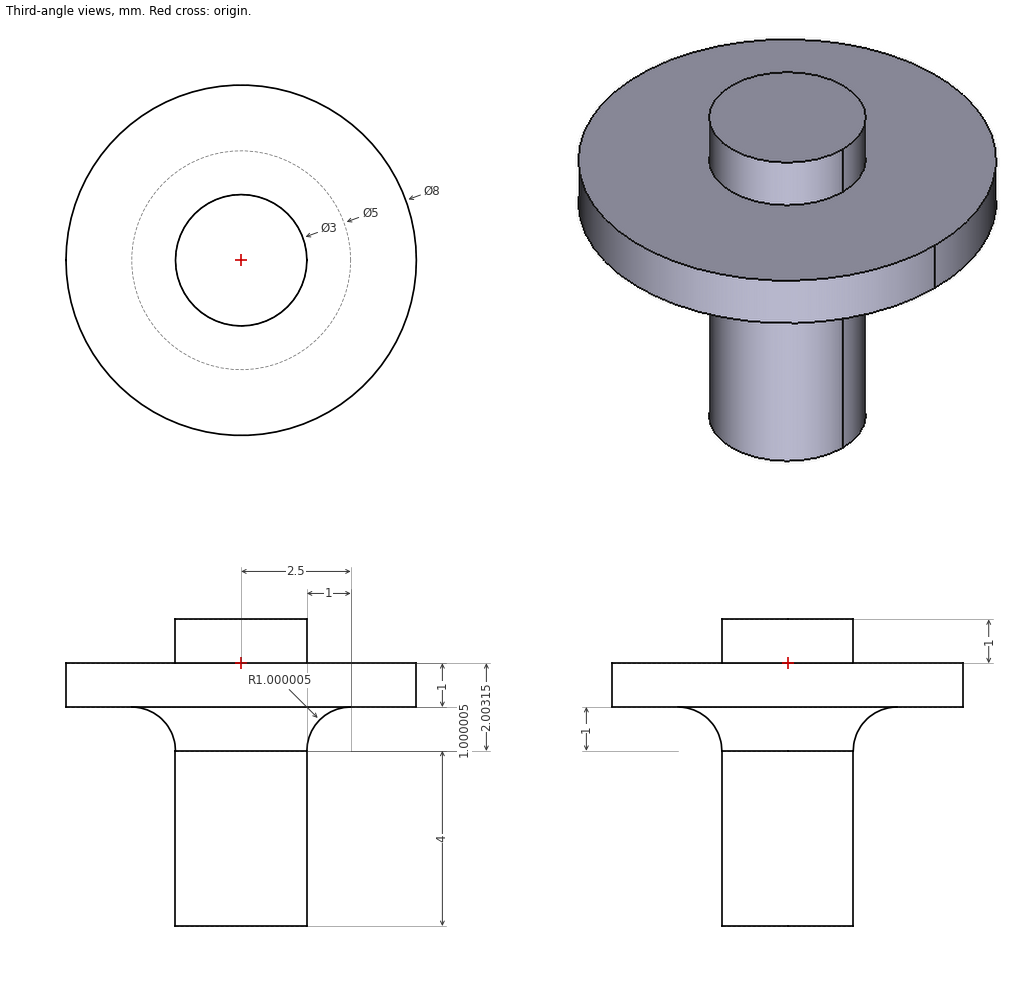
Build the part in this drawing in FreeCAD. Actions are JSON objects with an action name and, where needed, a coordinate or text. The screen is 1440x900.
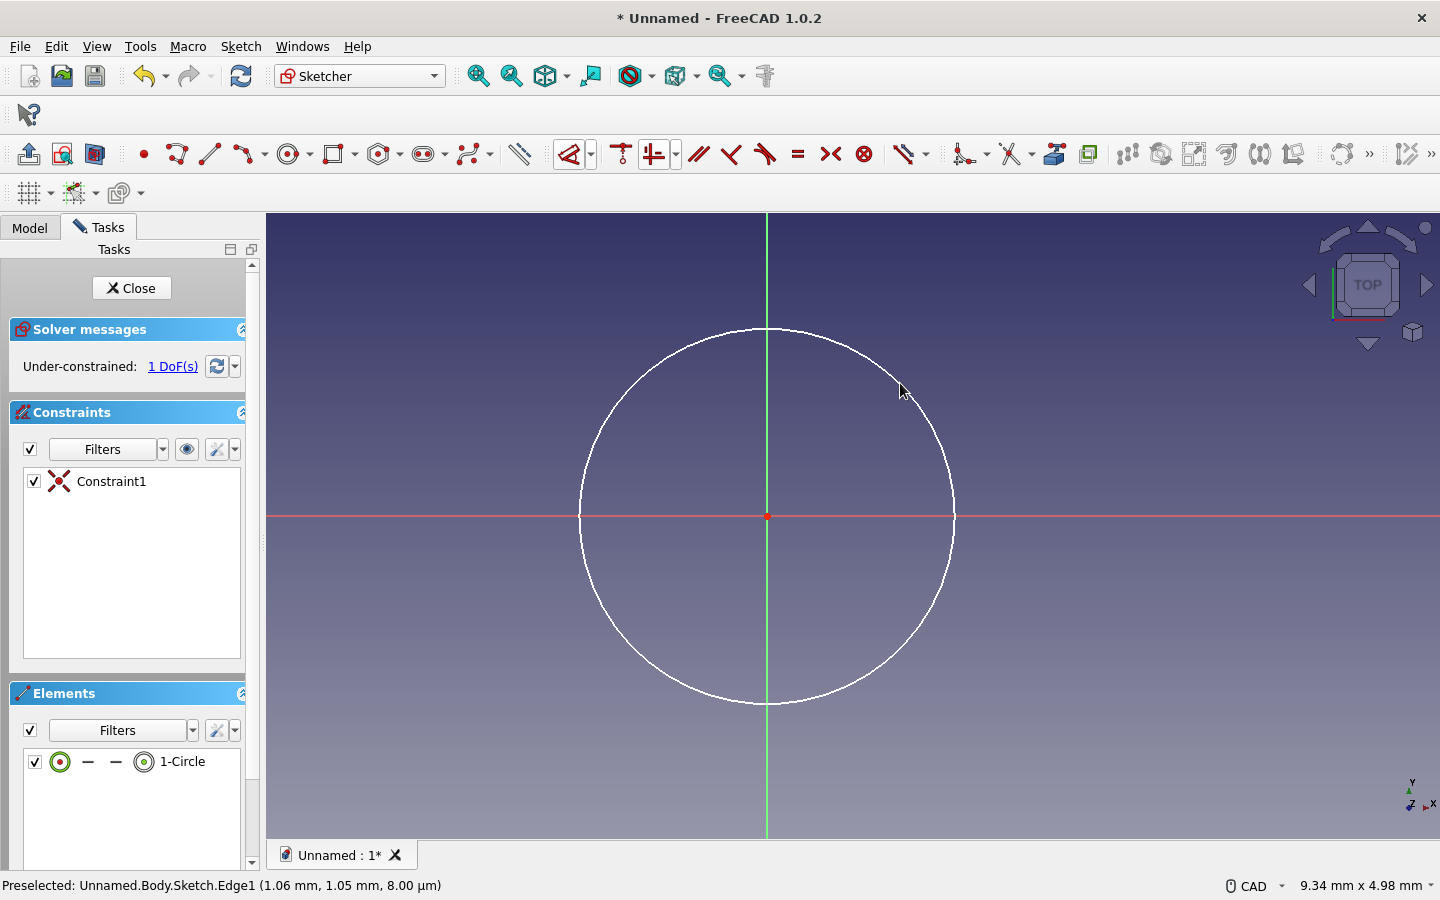
{"action": "left_click", "coordinate": [899, 383]}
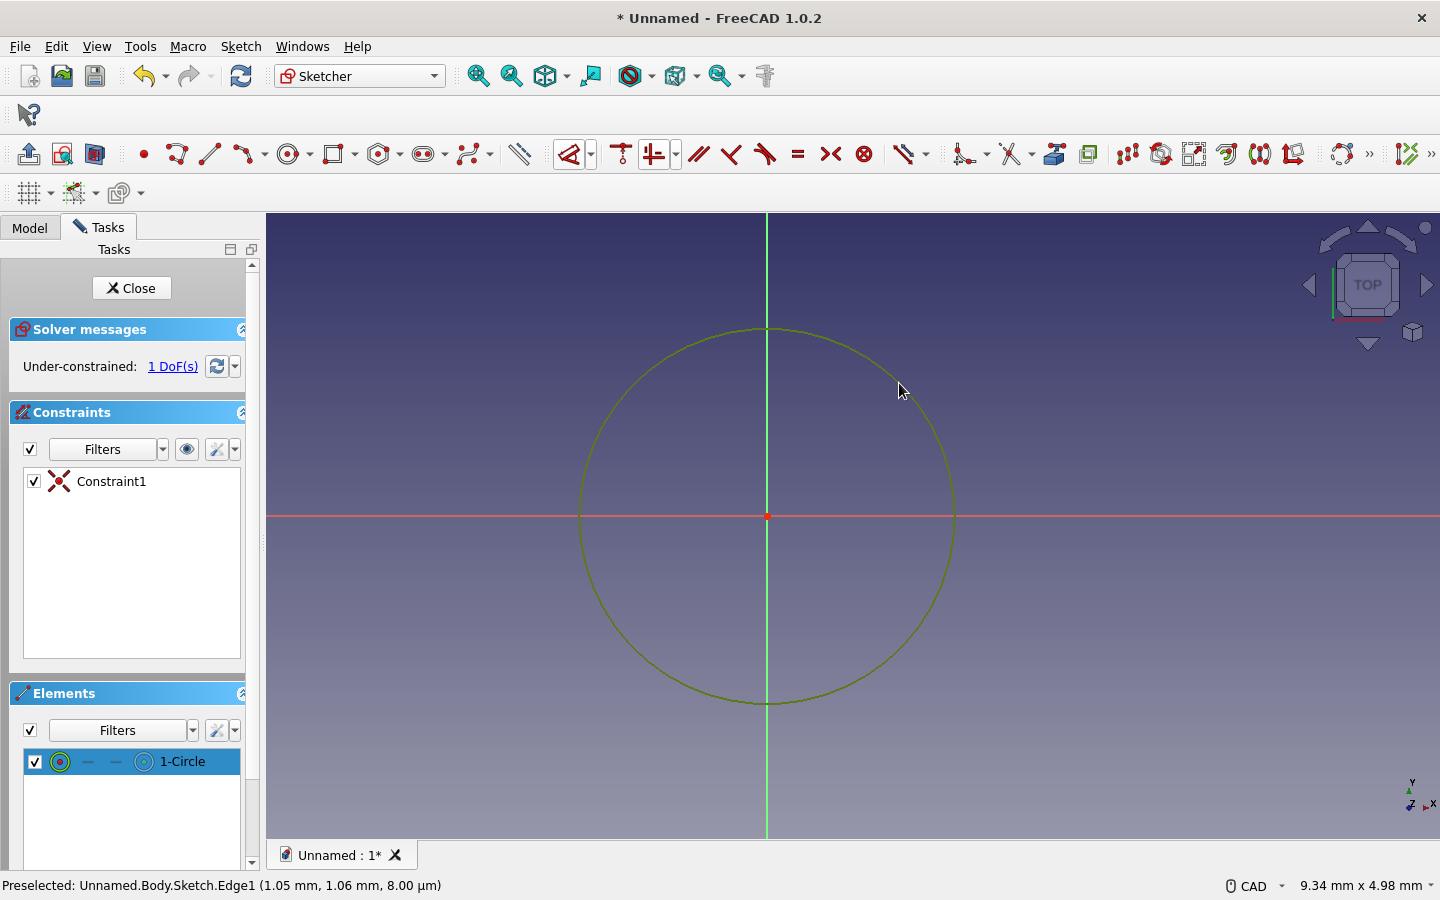
{"action": "key", "text": "k o"}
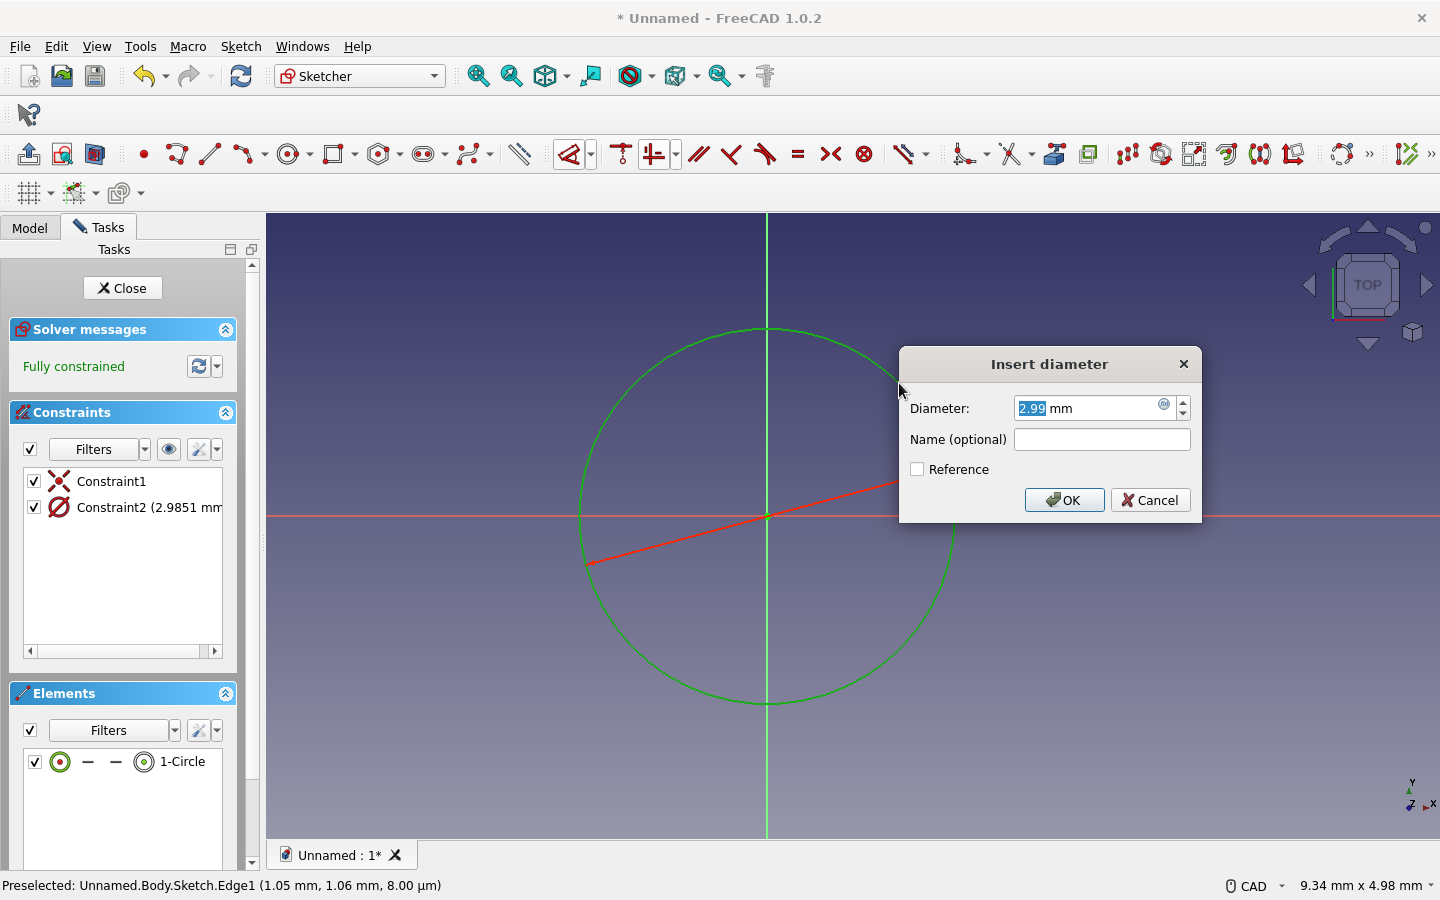
{"action": "type", "text": "3"}
{"action": "key", "text": "Return"}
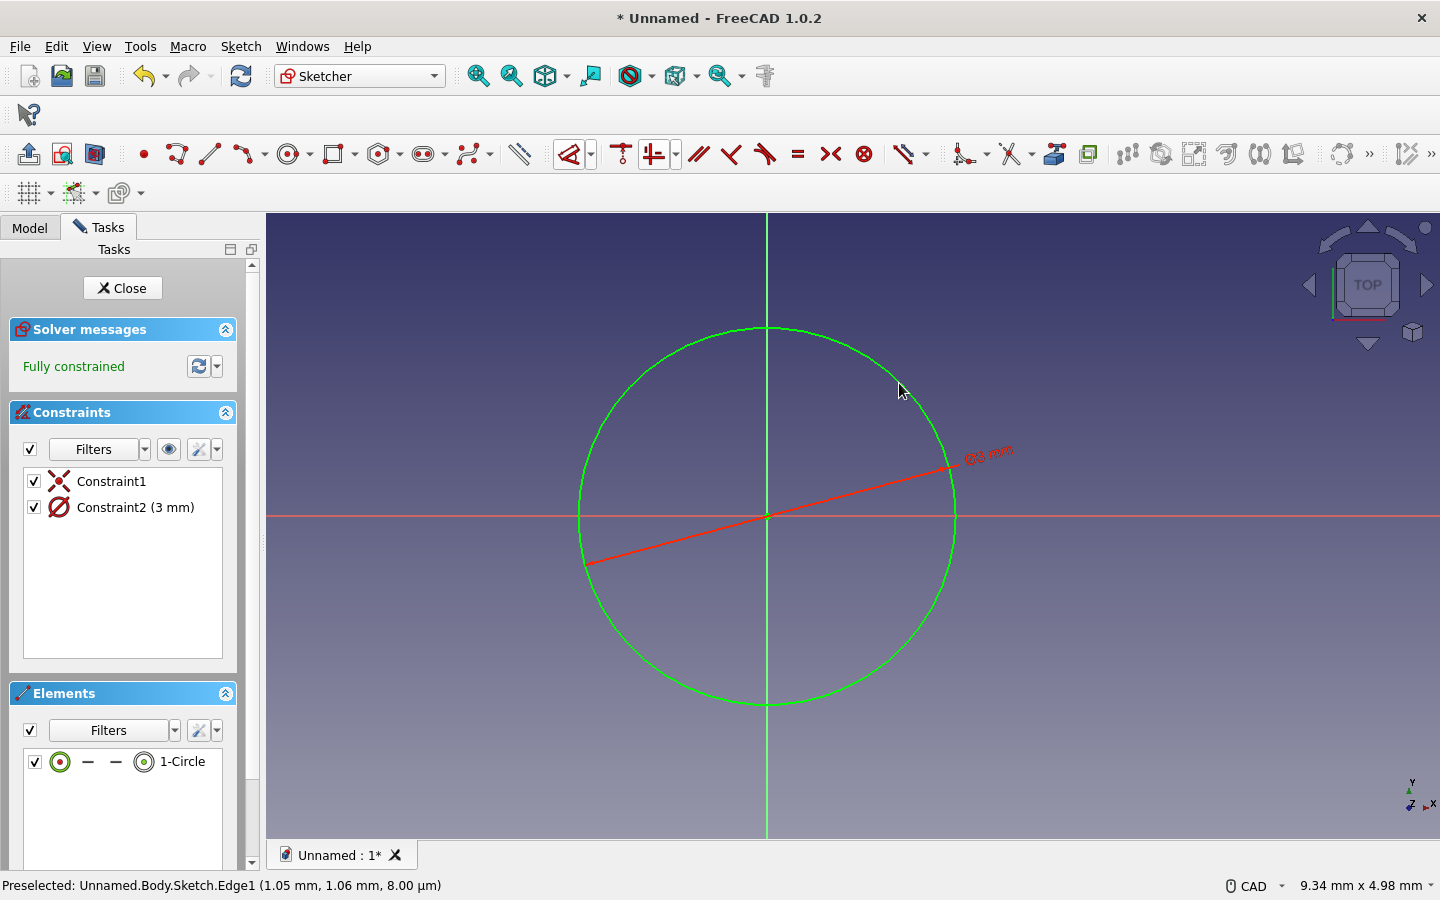
{"action": "left_click", "coordinate": [123, 288]}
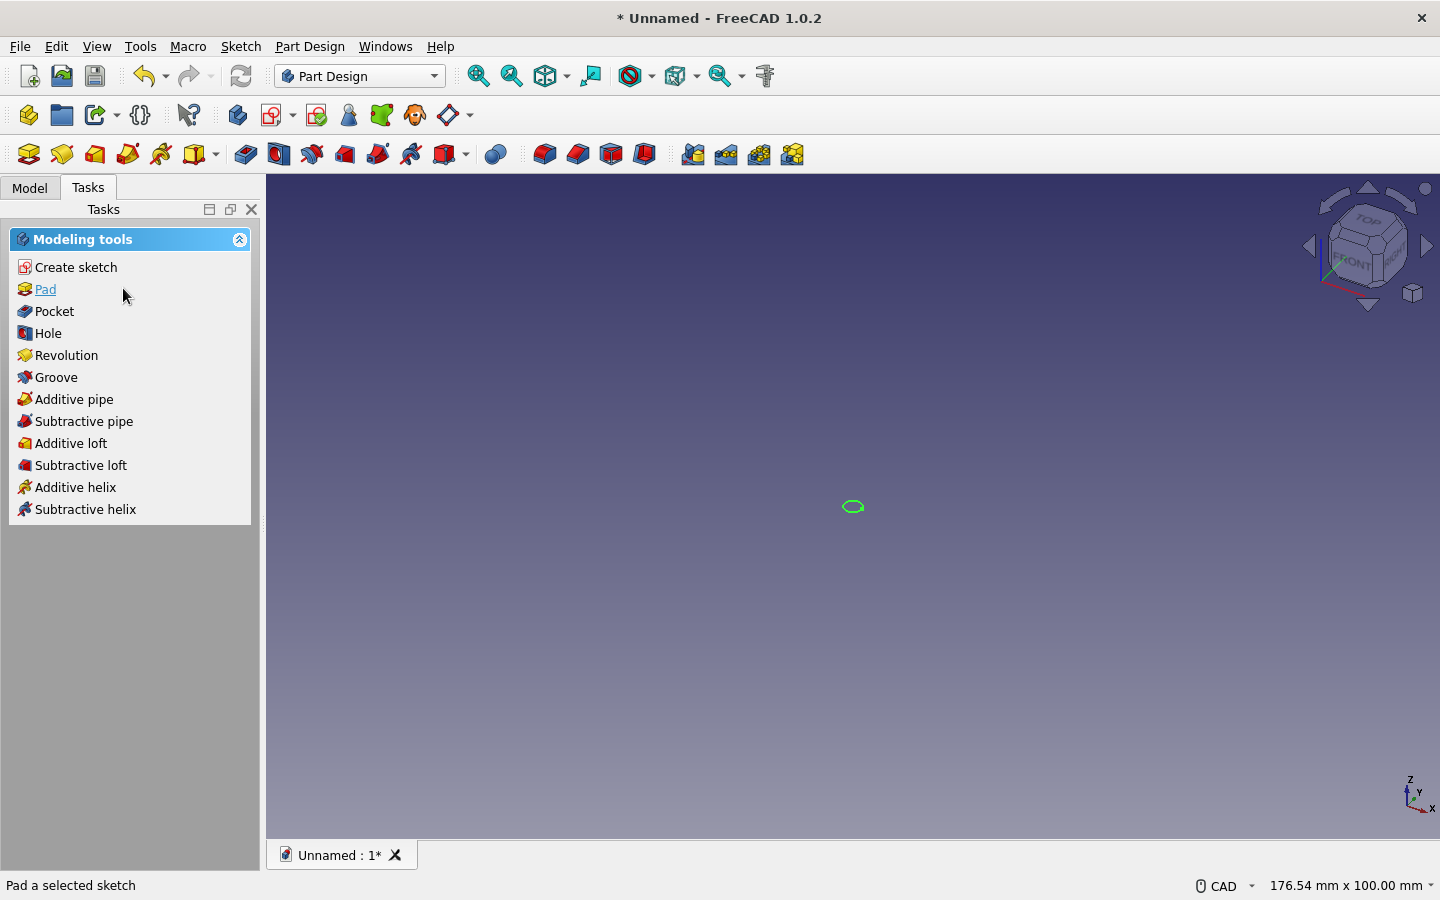
{"action": "left_click", "coordinate": [29, 154]}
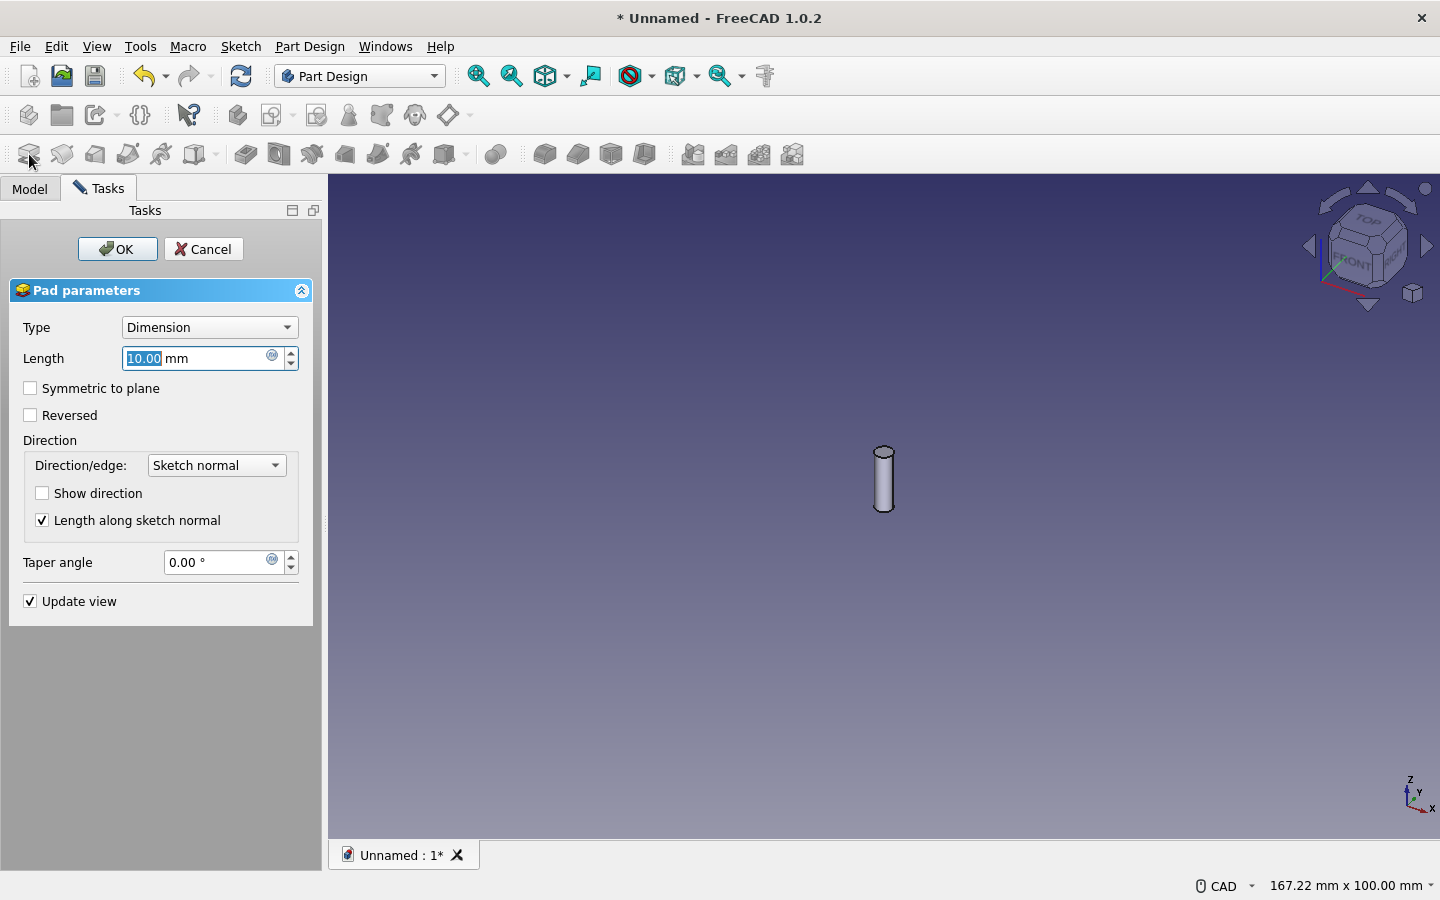
{"action": "type", "text": "1"}
{"action": "key", "text": "Tab"}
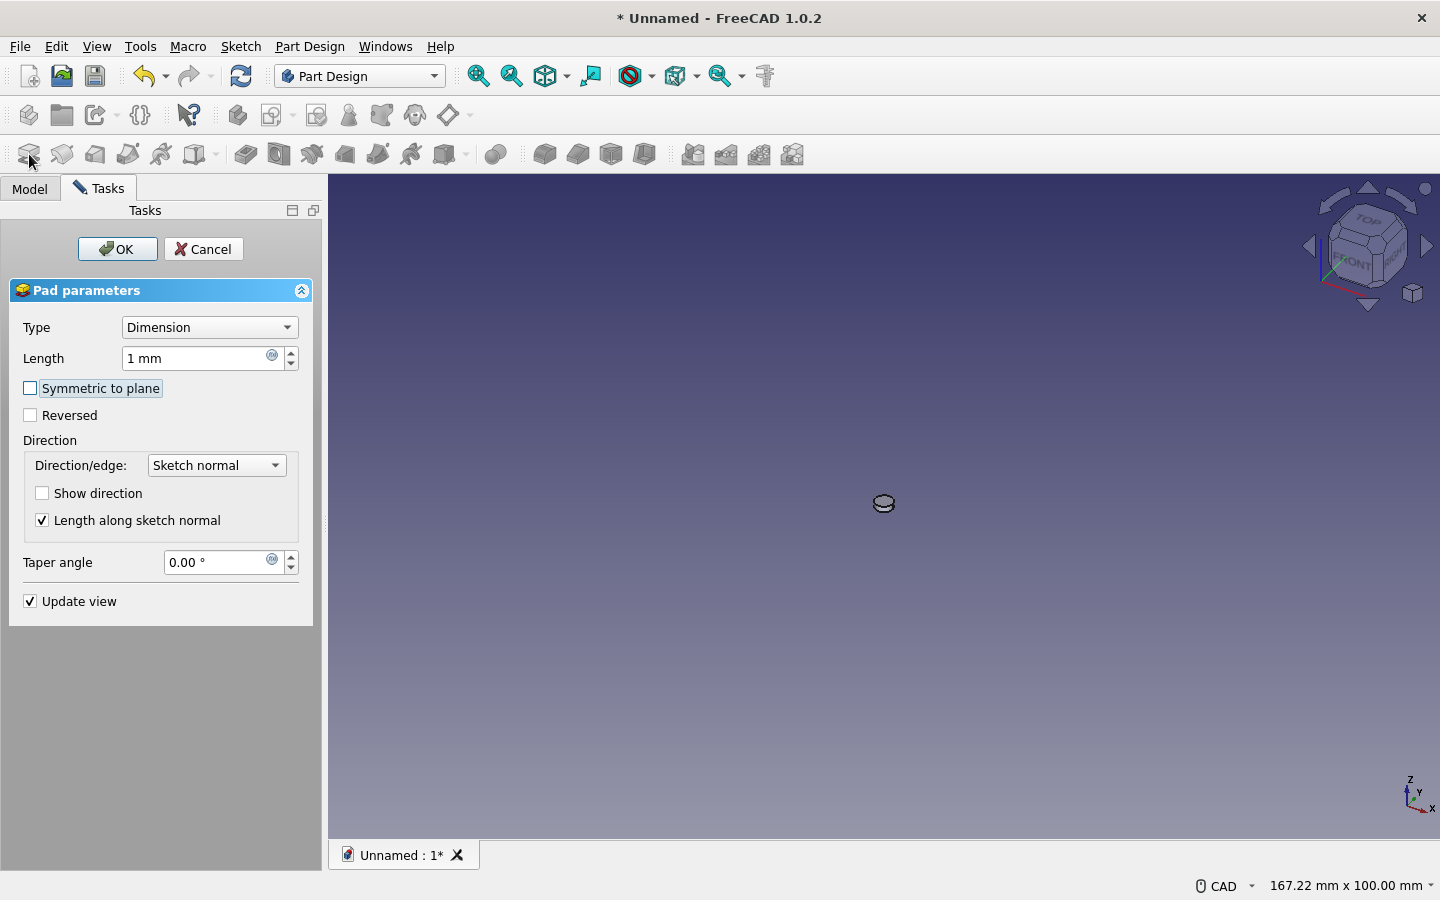
{"action": "left_click", "coordinate": [118, 249]}